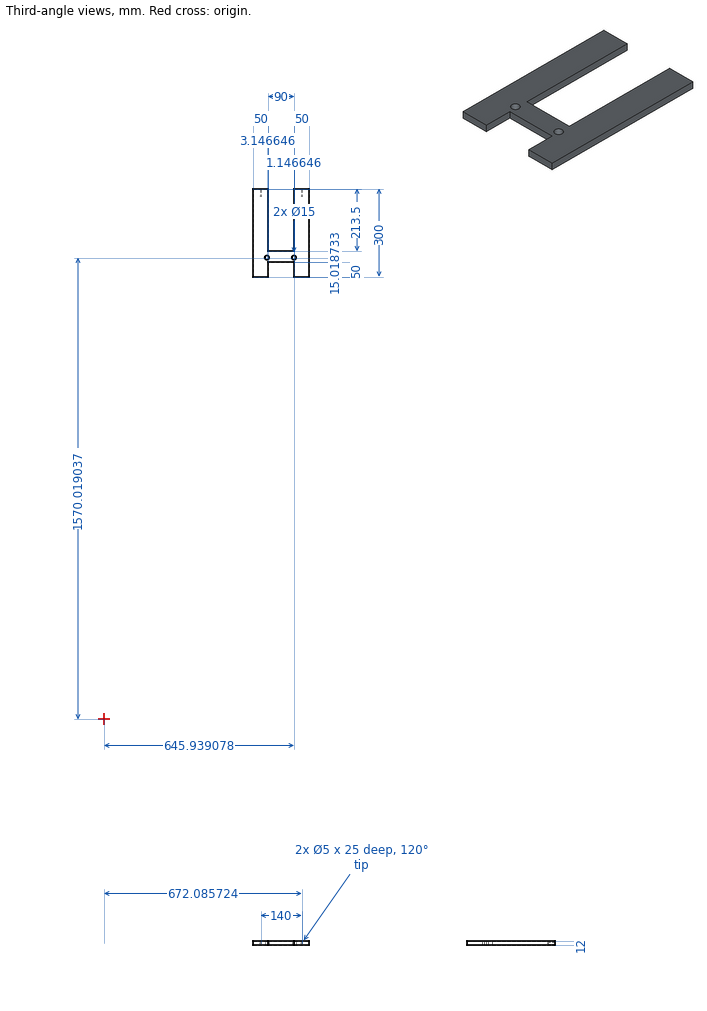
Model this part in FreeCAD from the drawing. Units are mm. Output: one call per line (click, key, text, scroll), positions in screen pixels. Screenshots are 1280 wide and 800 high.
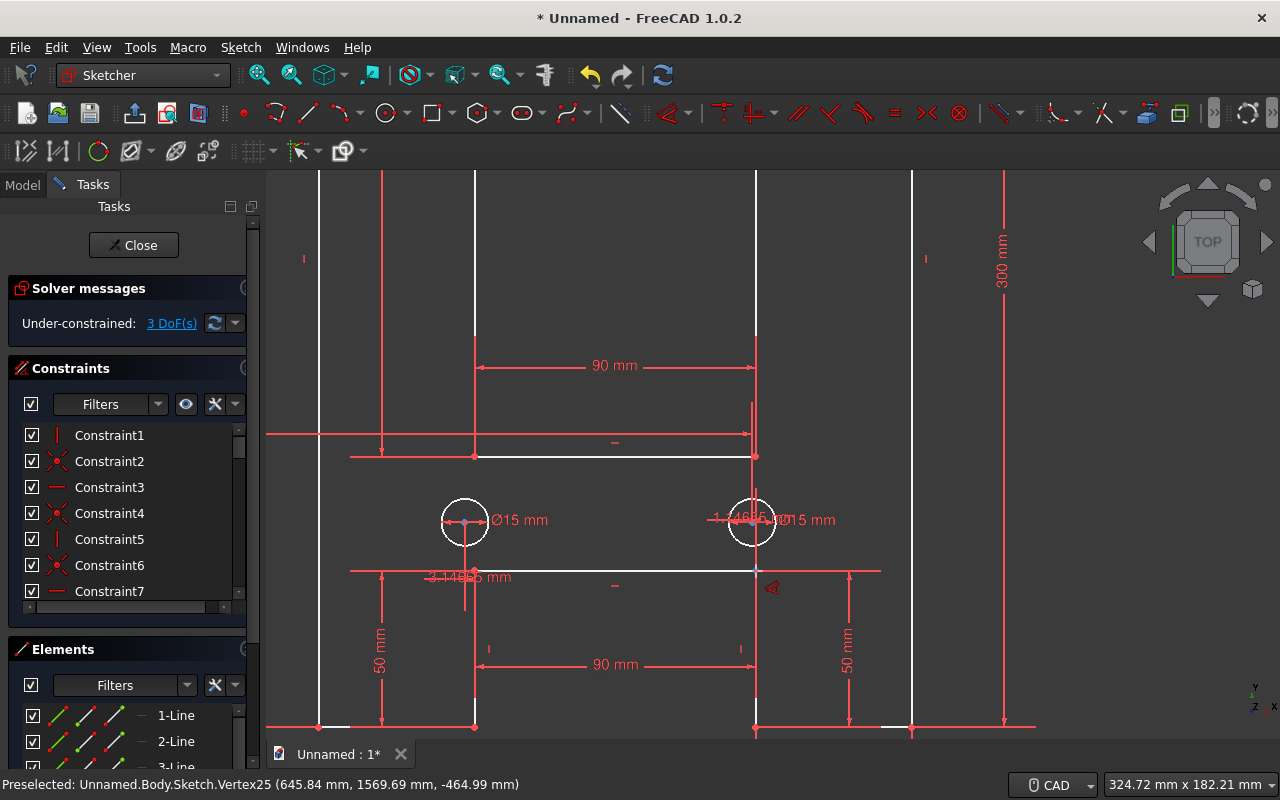
click(756, 571)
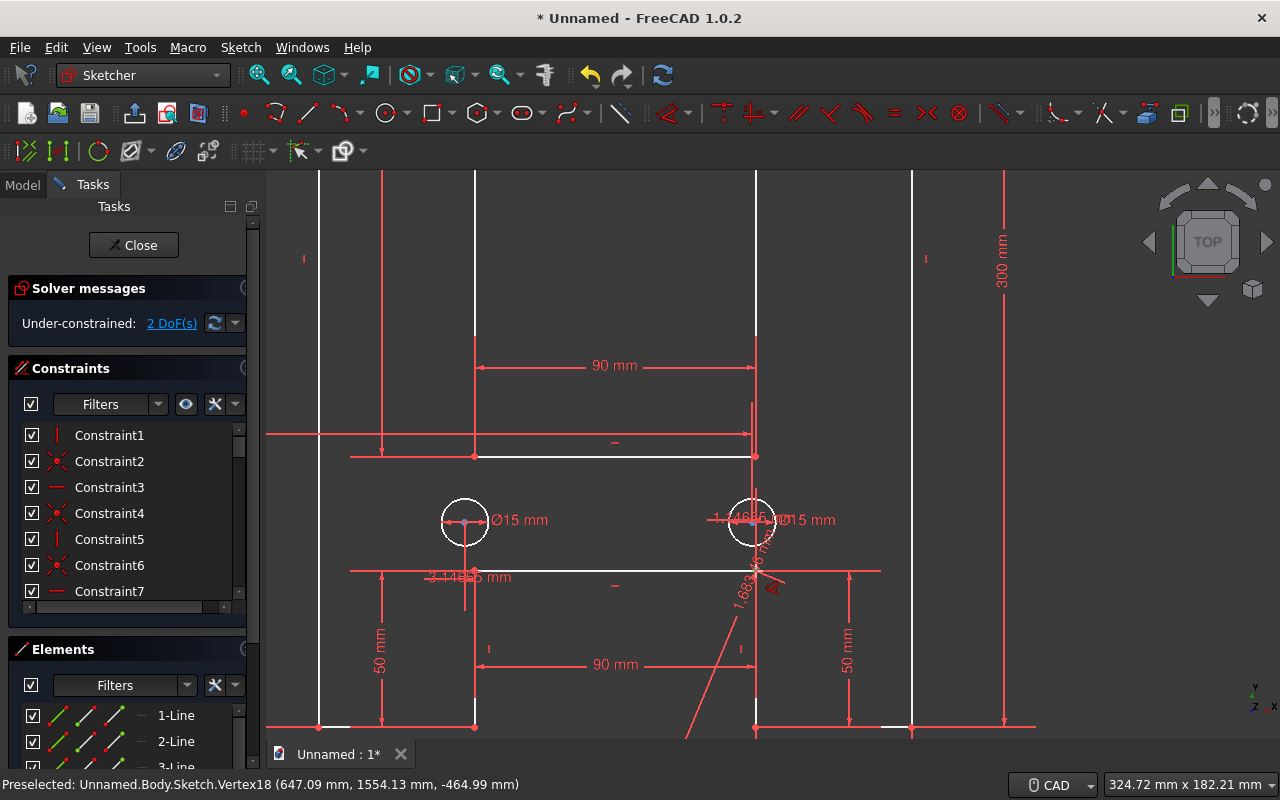
click(752, 522)
click(790, 547)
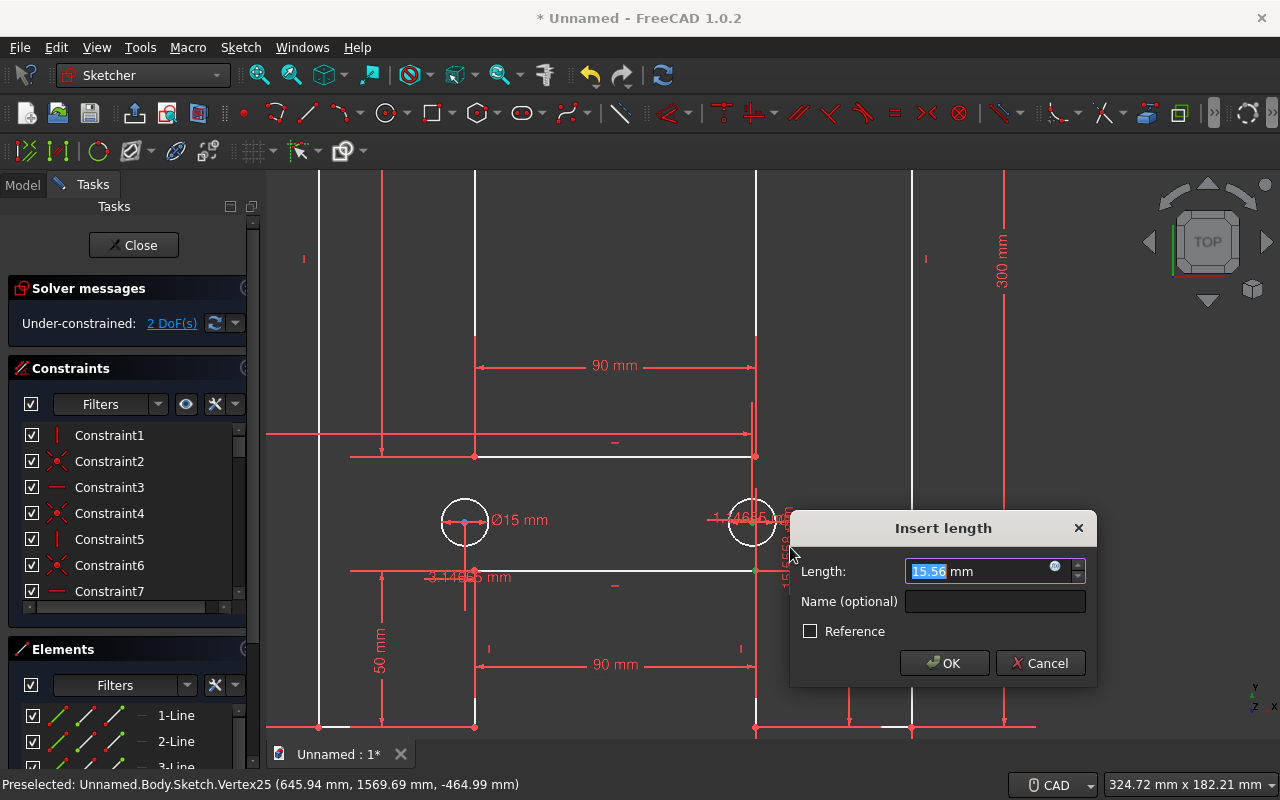
text(15.018733)
key(Return)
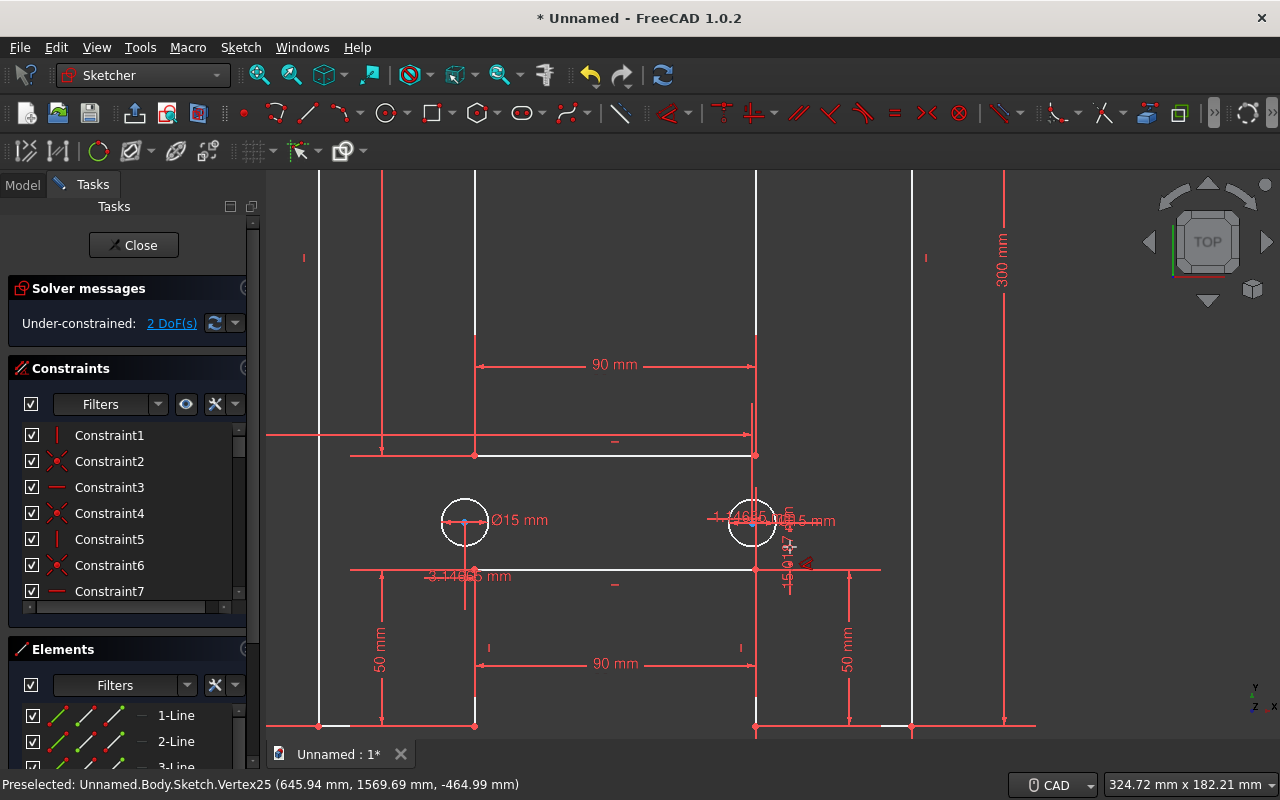
click(475, 570)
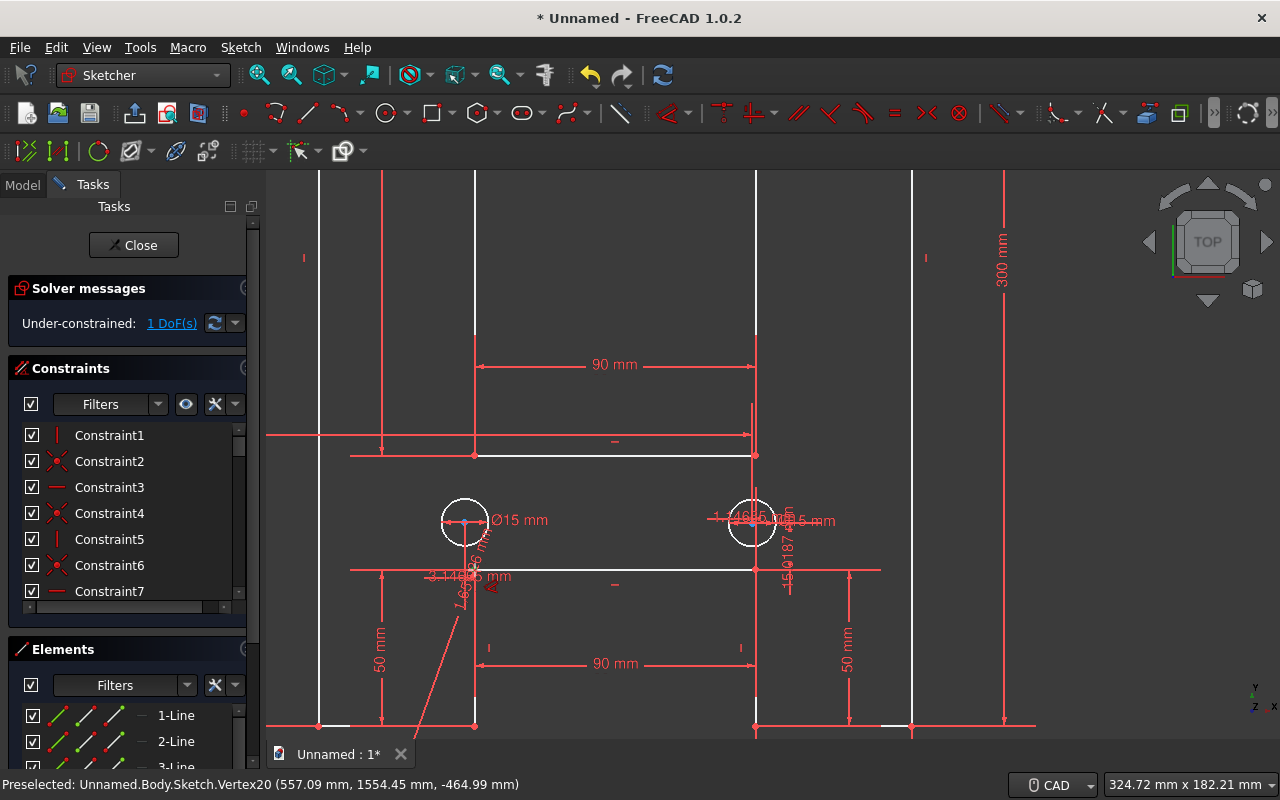
click(465, 522)
click(431, 546)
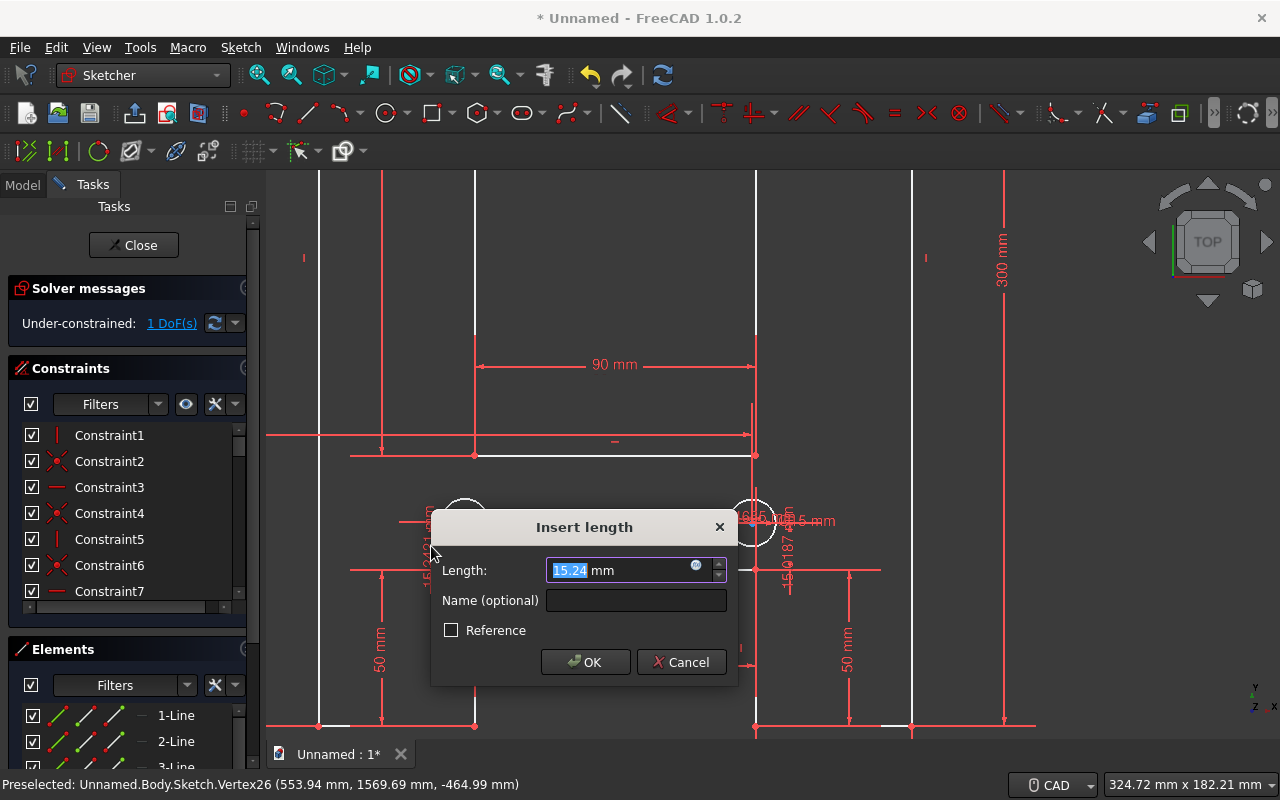
text(15.018733)
key(Return)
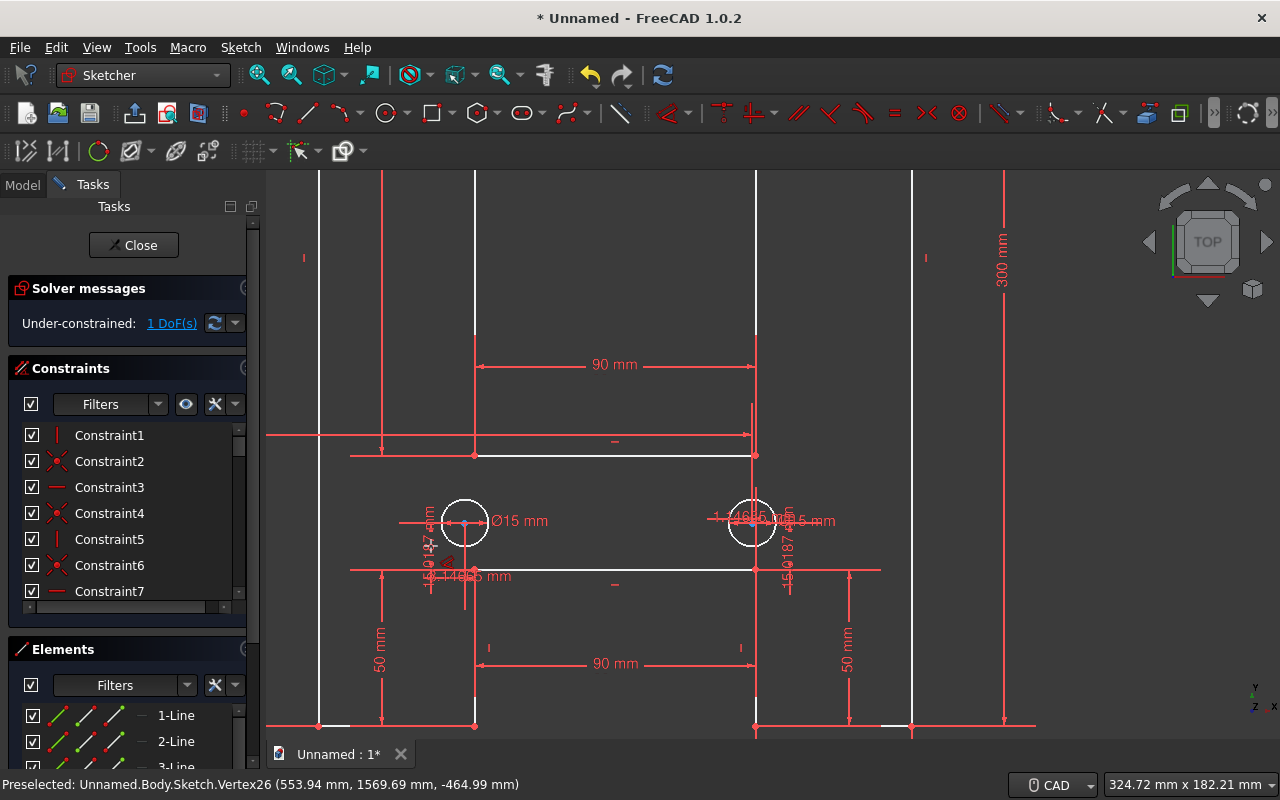
click(752, 523)
click(786, 617)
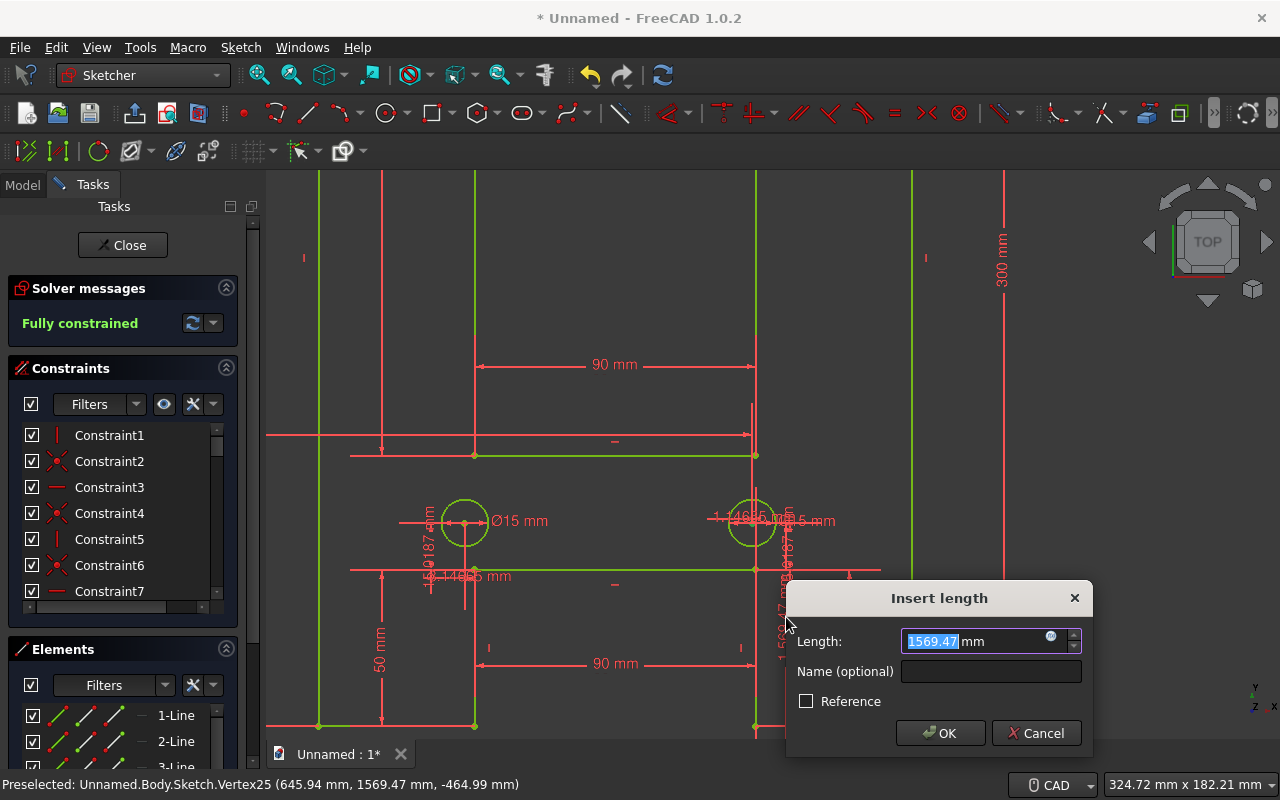
text(1570.019037)
key(Return)
key(Escape)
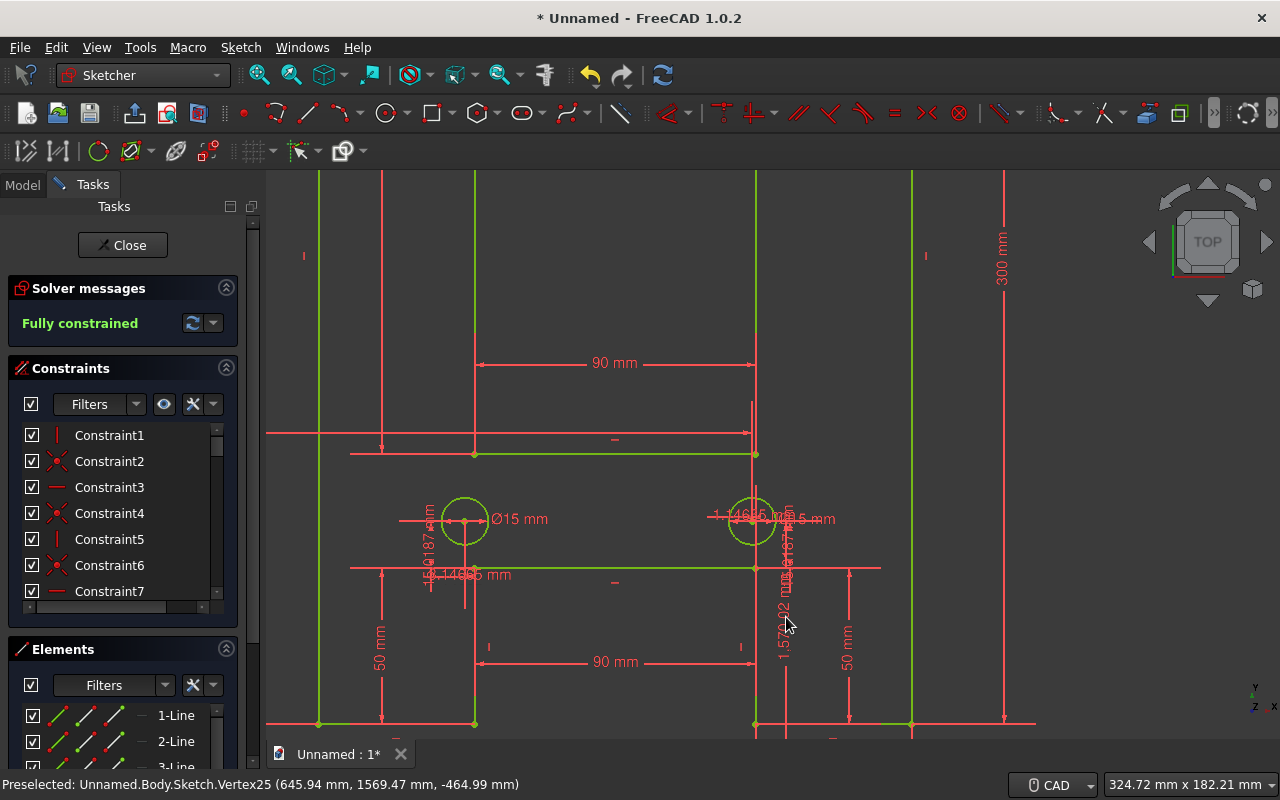
click(123, 245)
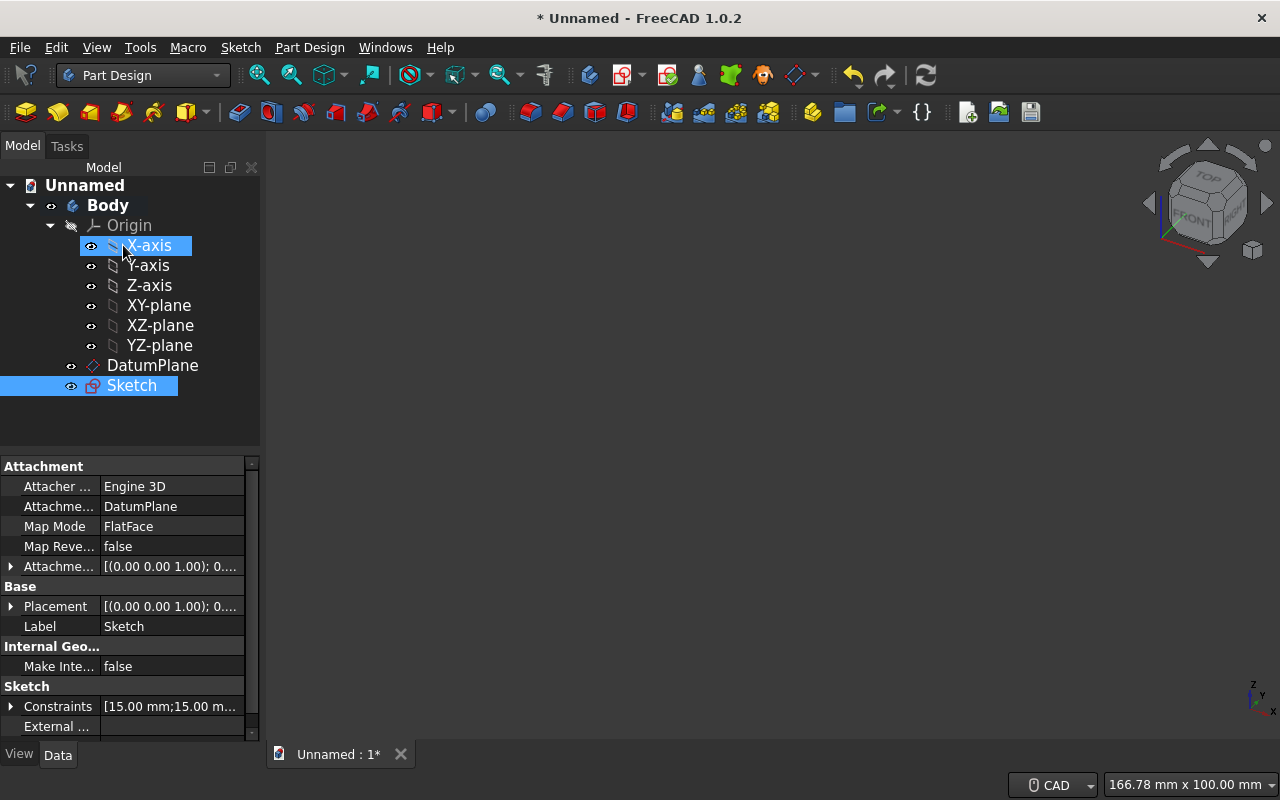
click(26, 112)